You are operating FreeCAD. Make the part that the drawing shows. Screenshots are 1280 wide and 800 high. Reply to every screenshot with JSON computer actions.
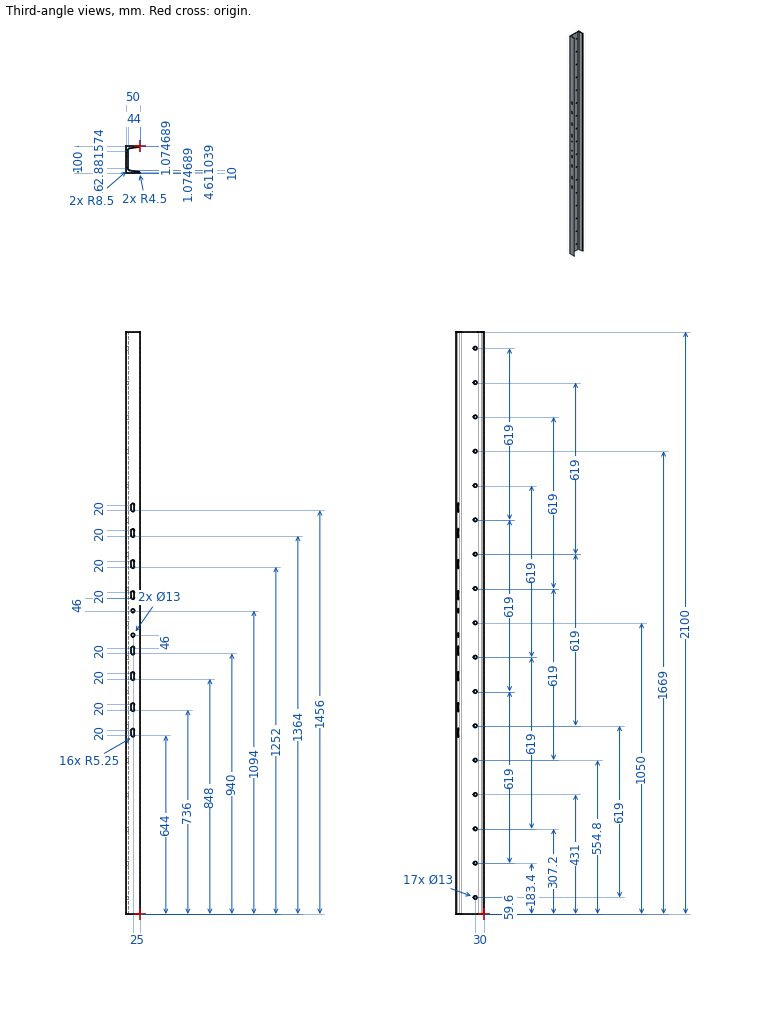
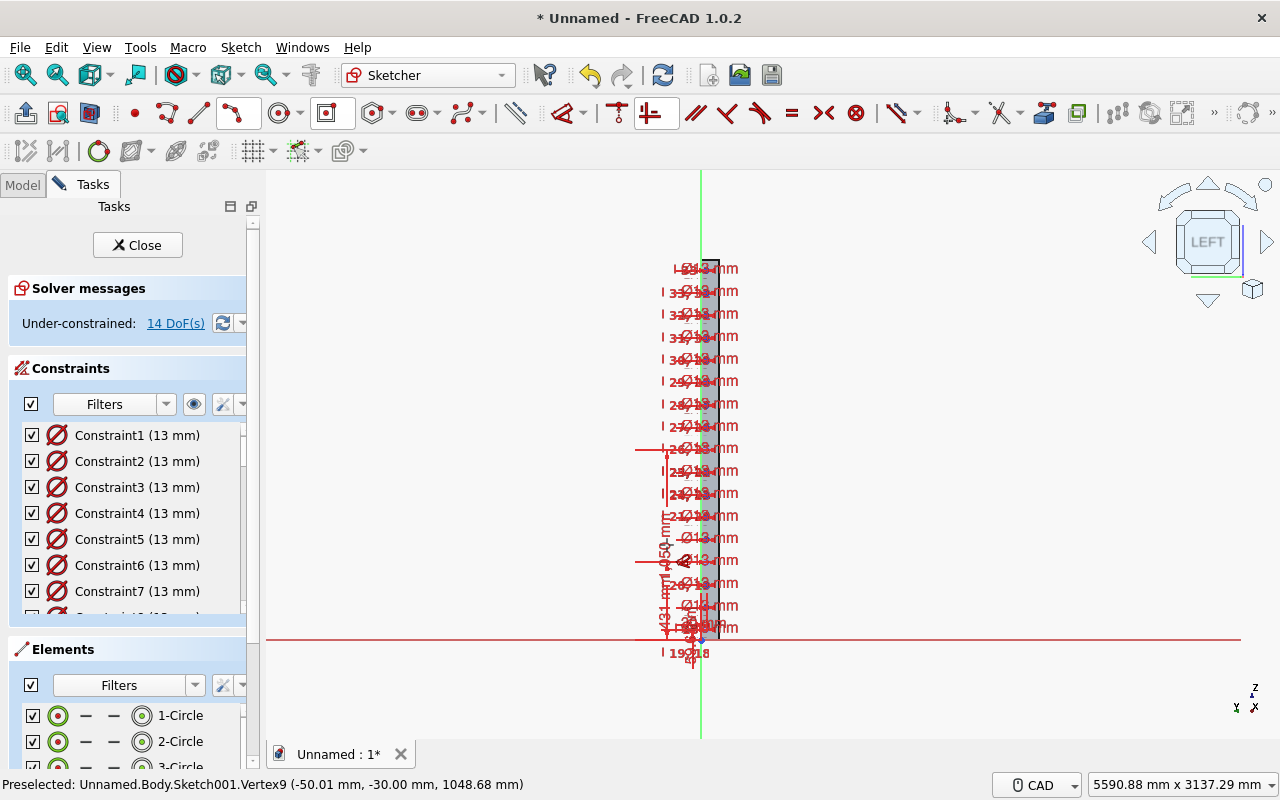
{"action": "left_click", "coordinate": [707, 338]}
{"action": "left_click", "coordinate": [667, 489]}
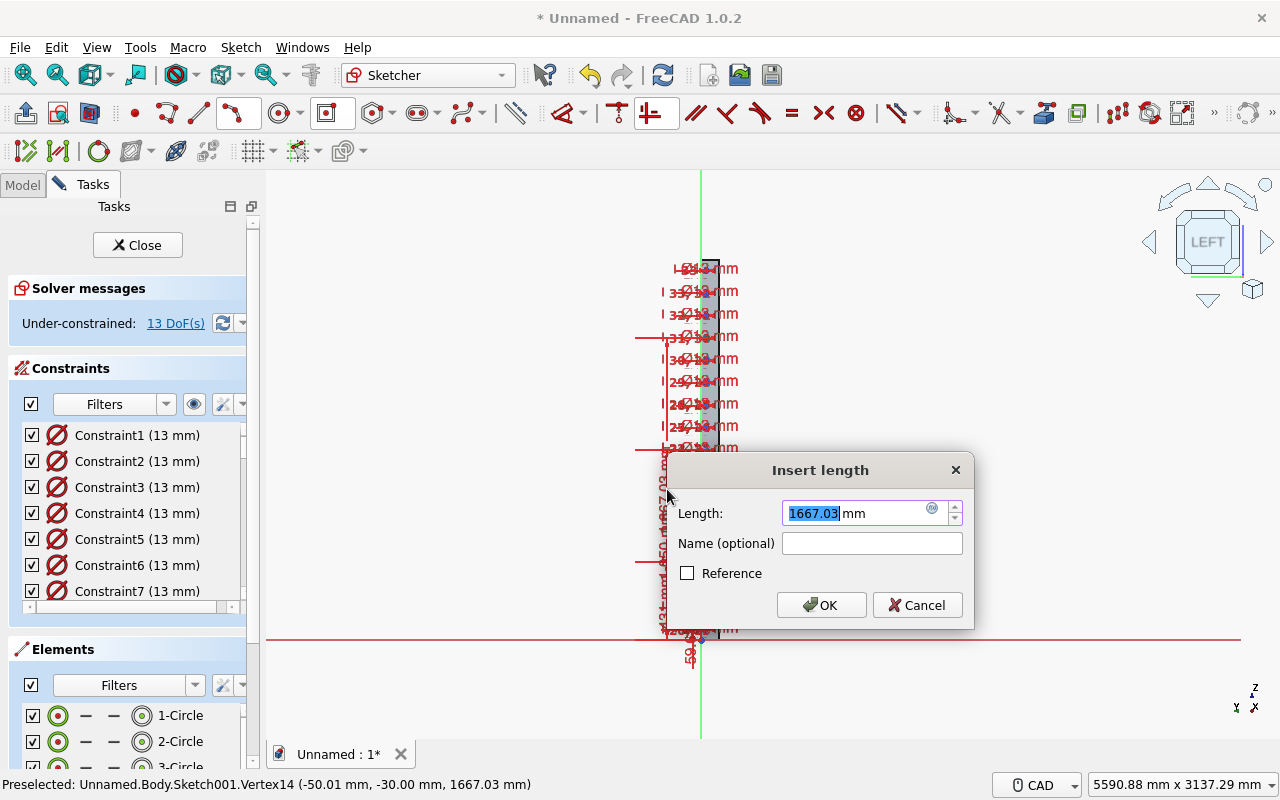
{"action": "type", "text": "1669"}
{"action": "key", "text": "Return"}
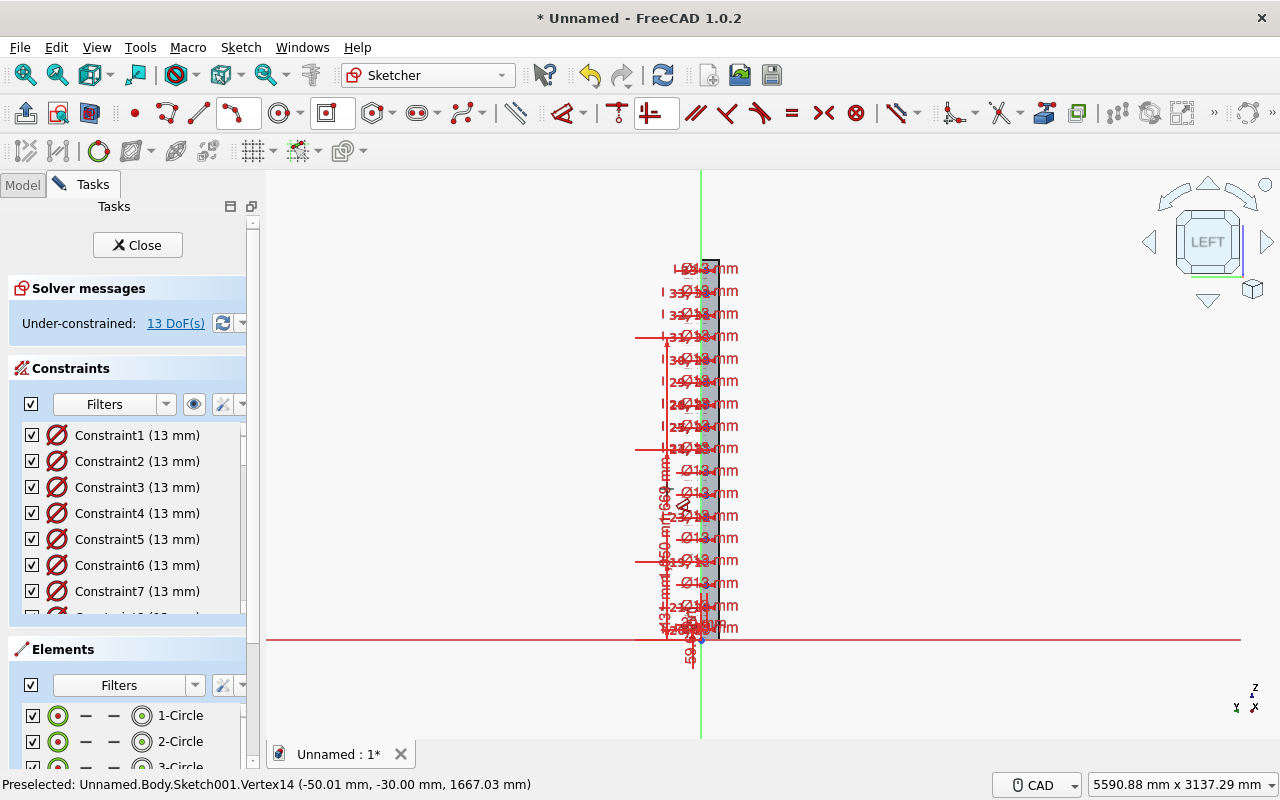
{"action": "left_click", "coordinate": [707, 630]}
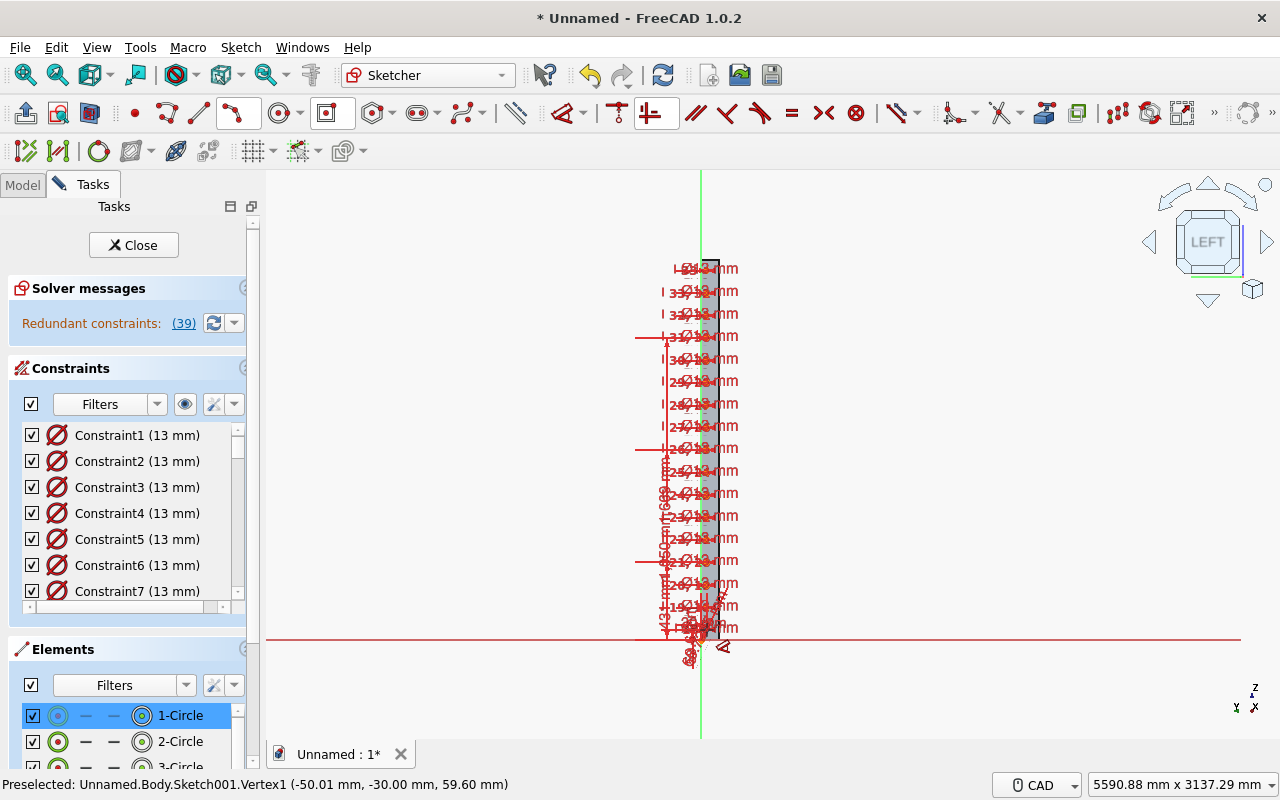
{"action": "left_click", "coordinate": [707, 518]}
{"action": "left_click", "coordinate": [741, 574]}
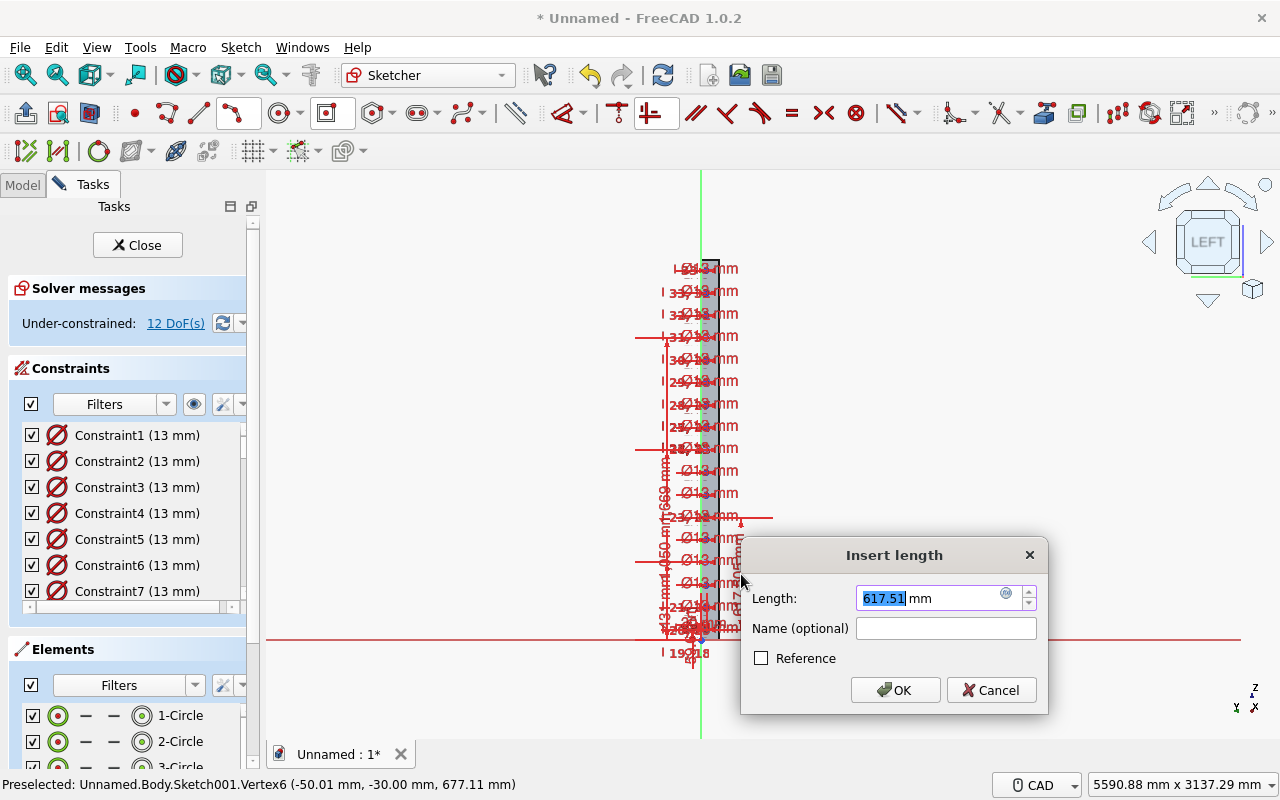
{"action": "type", "text": "619"}
{"action": "key", "text": "Return"}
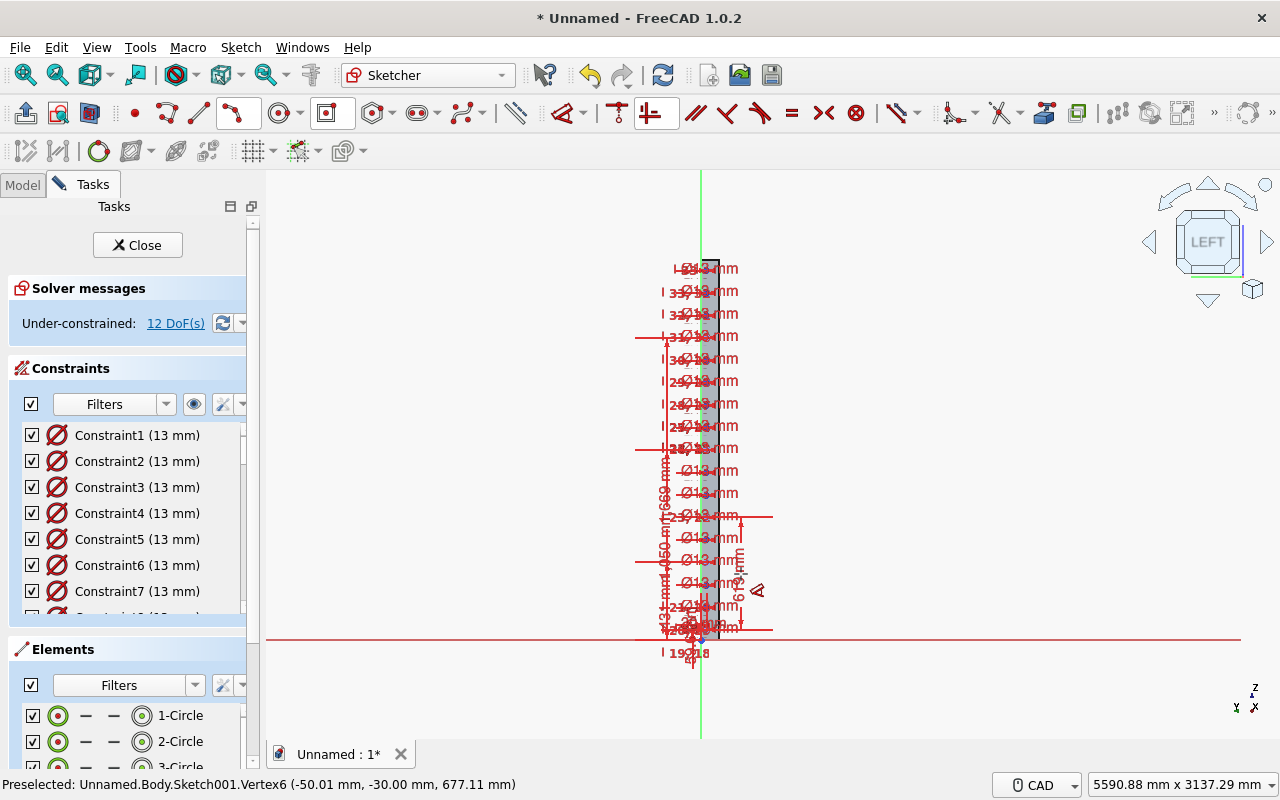
{"action": "left_click", "coordinate": [707, 608]}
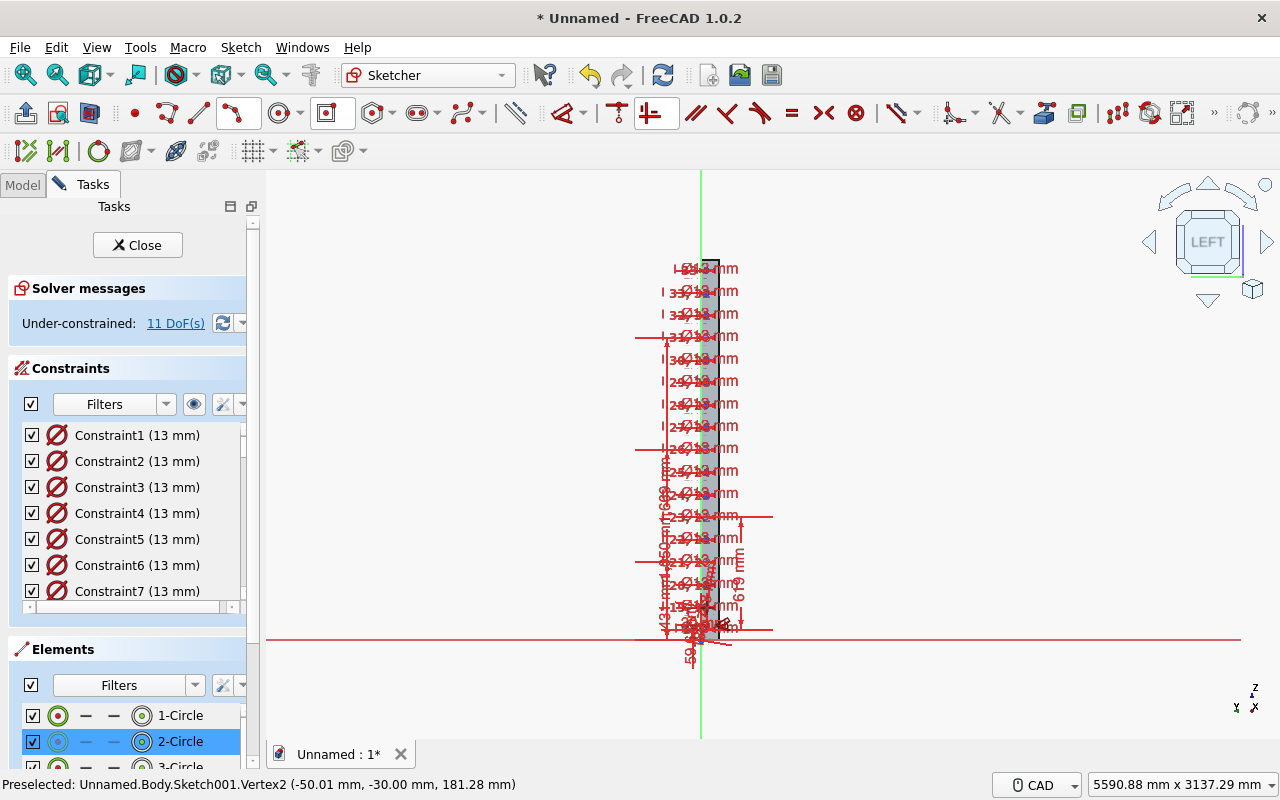
{"action": "left_click", "coordinate": [707, 495]}
{"action": "left_click", "coordinate": [741, 551]}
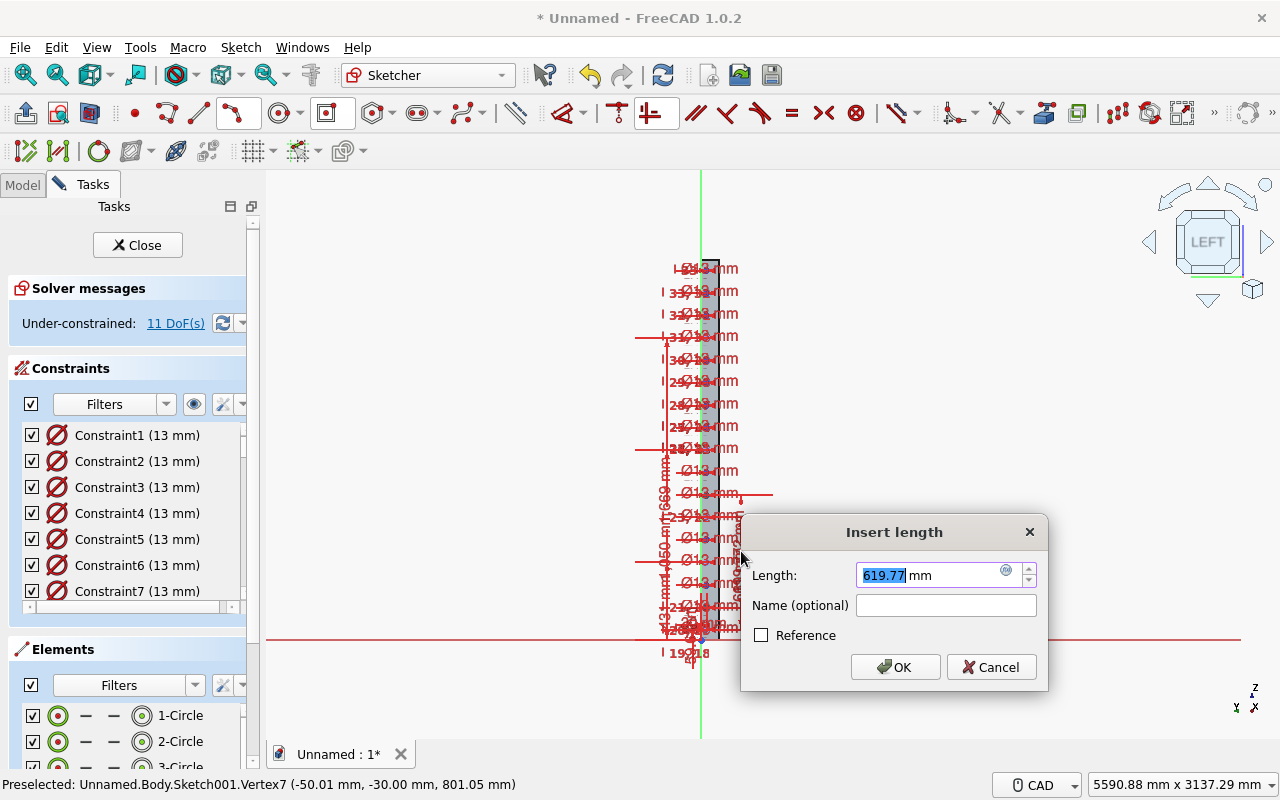
{"action": "type", "text": "619"}
{"action": "key", "text": "Return"}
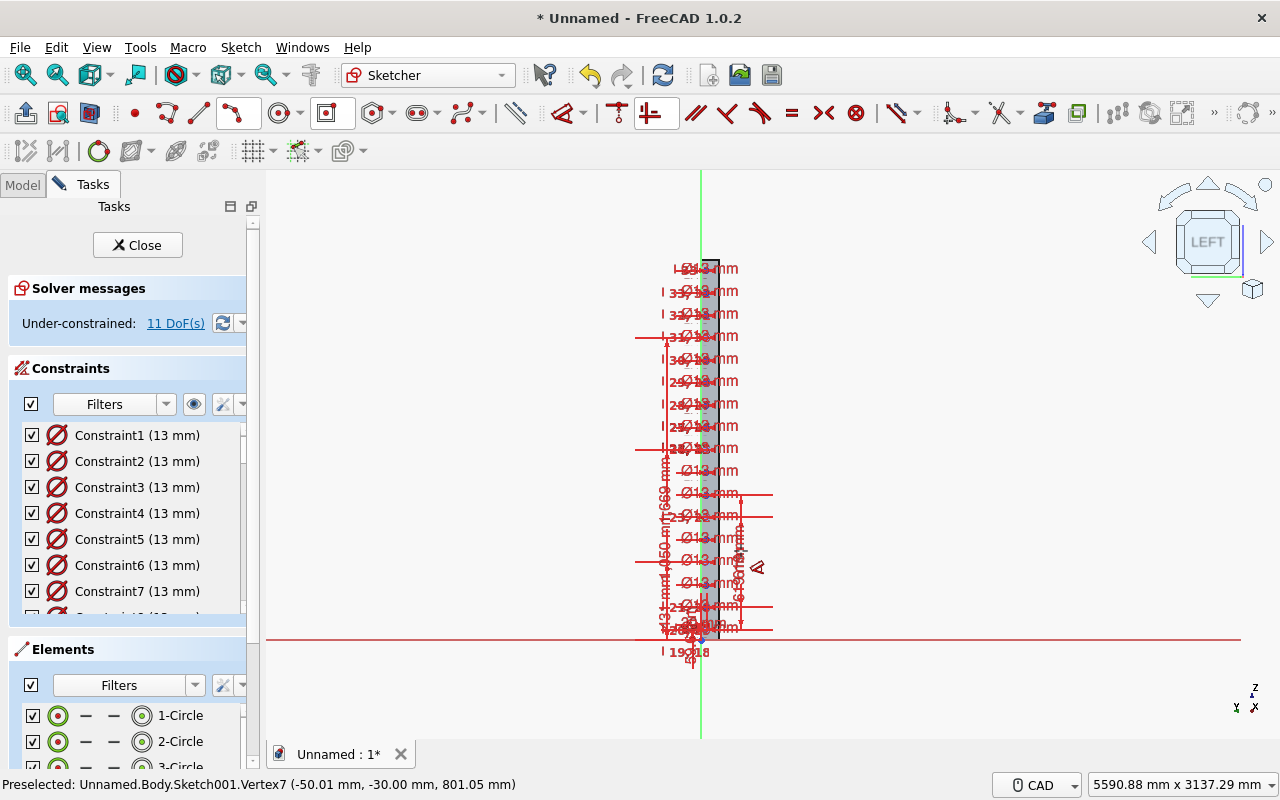
{"action": "left_click", "coordinate": [707, 585]}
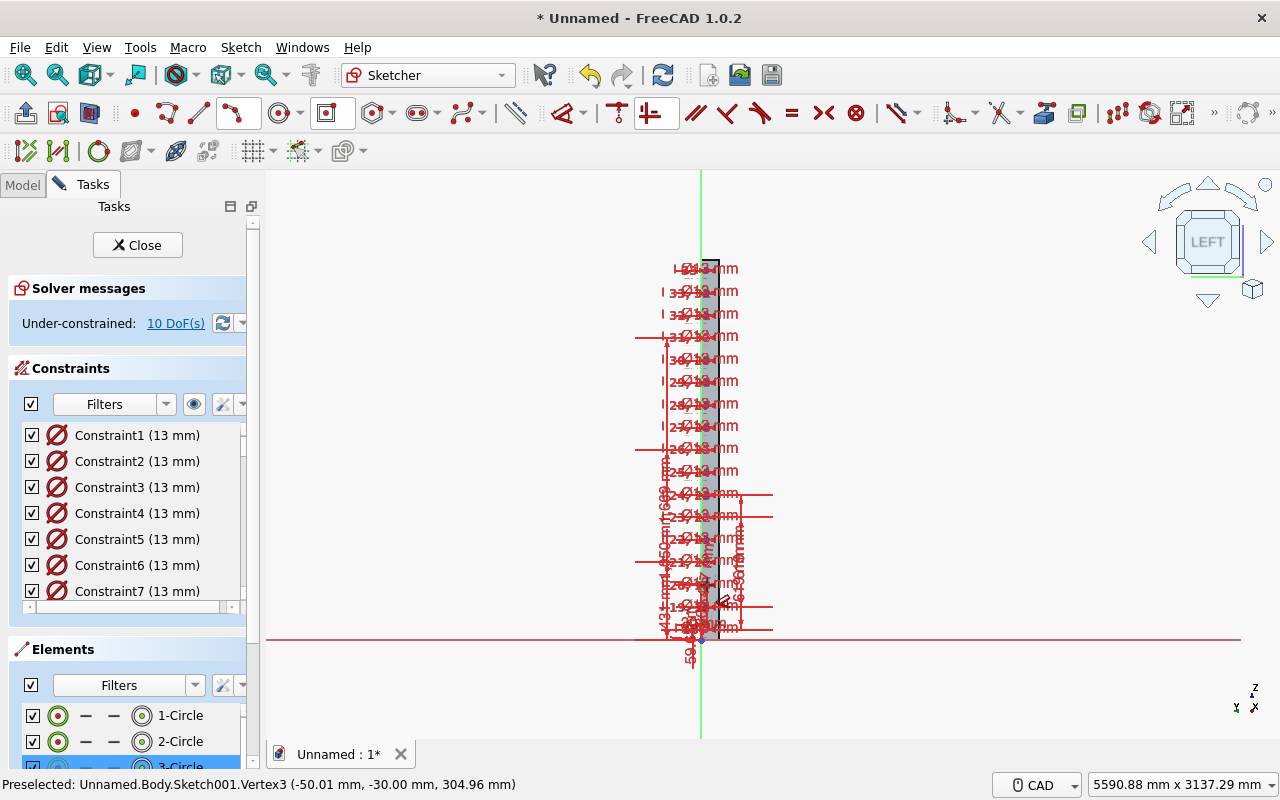
{"action": "left_click", "coordinate": [707, 473]}
{"action": "left_click", "coordinate": [741, 529]}